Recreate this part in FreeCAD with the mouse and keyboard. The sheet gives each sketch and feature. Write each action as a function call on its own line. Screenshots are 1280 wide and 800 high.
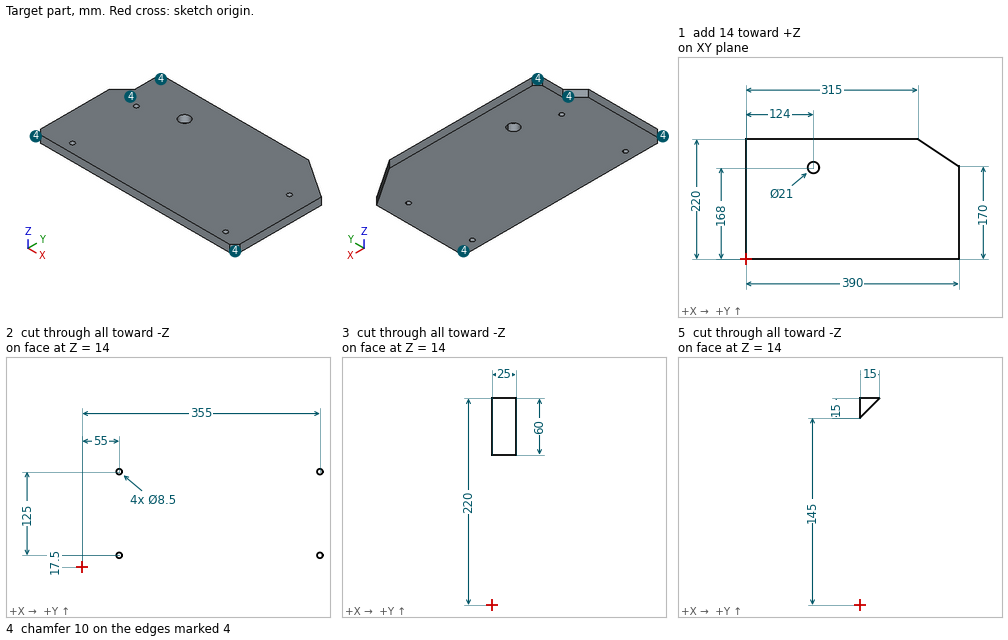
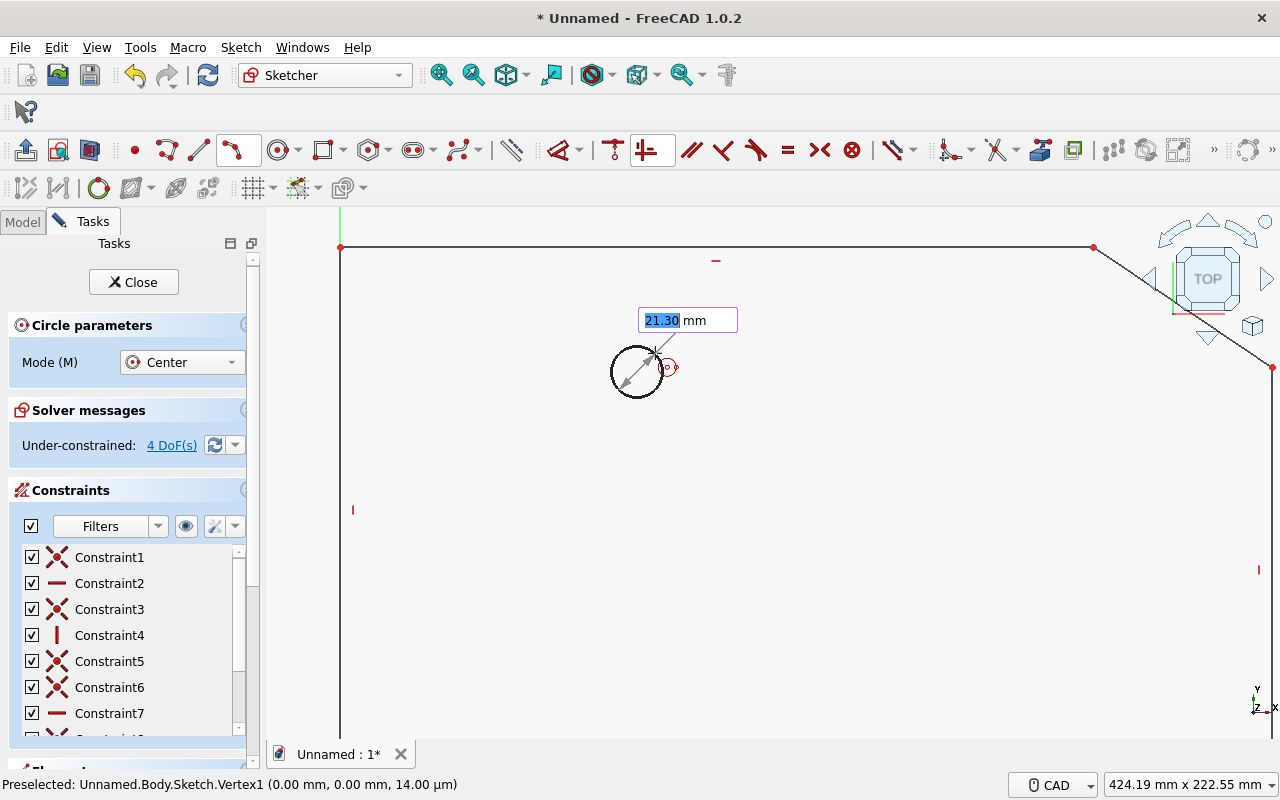
text(21)
key(Return)
key(Escape)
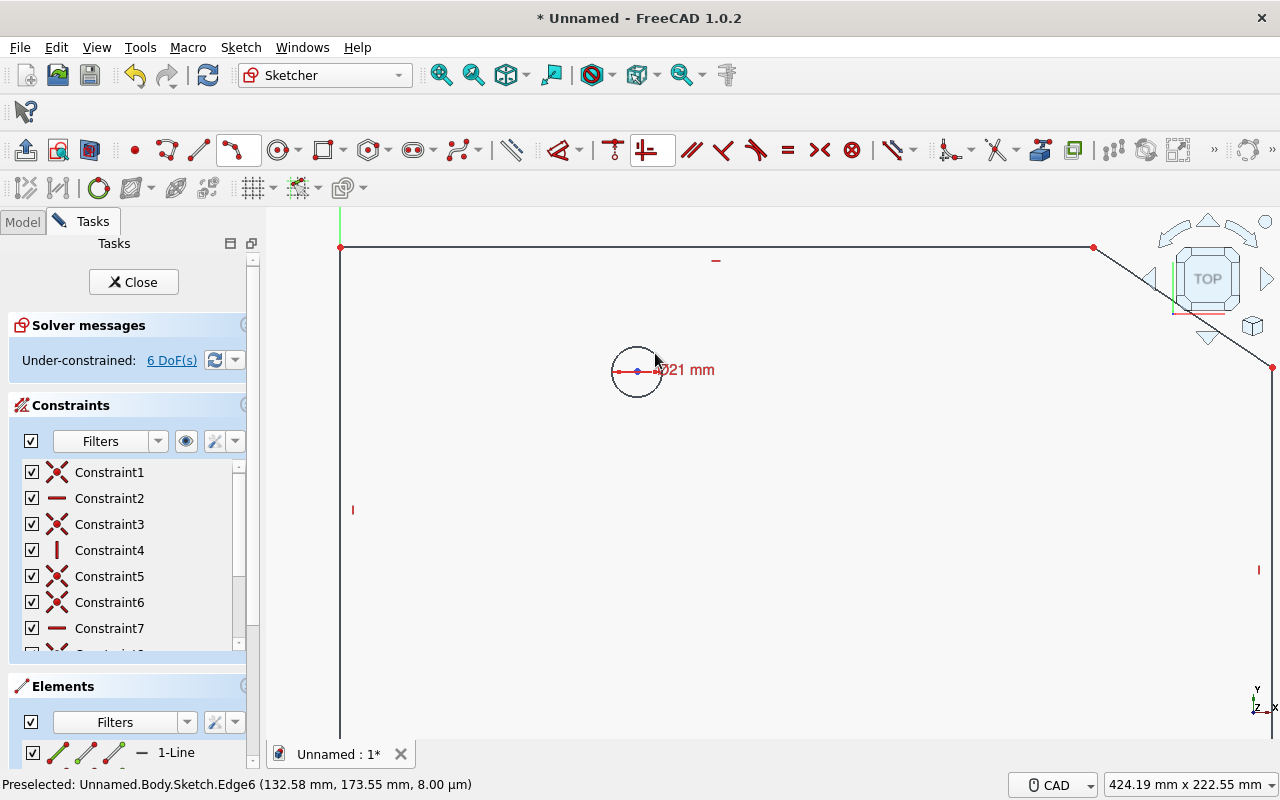
click(558, 150)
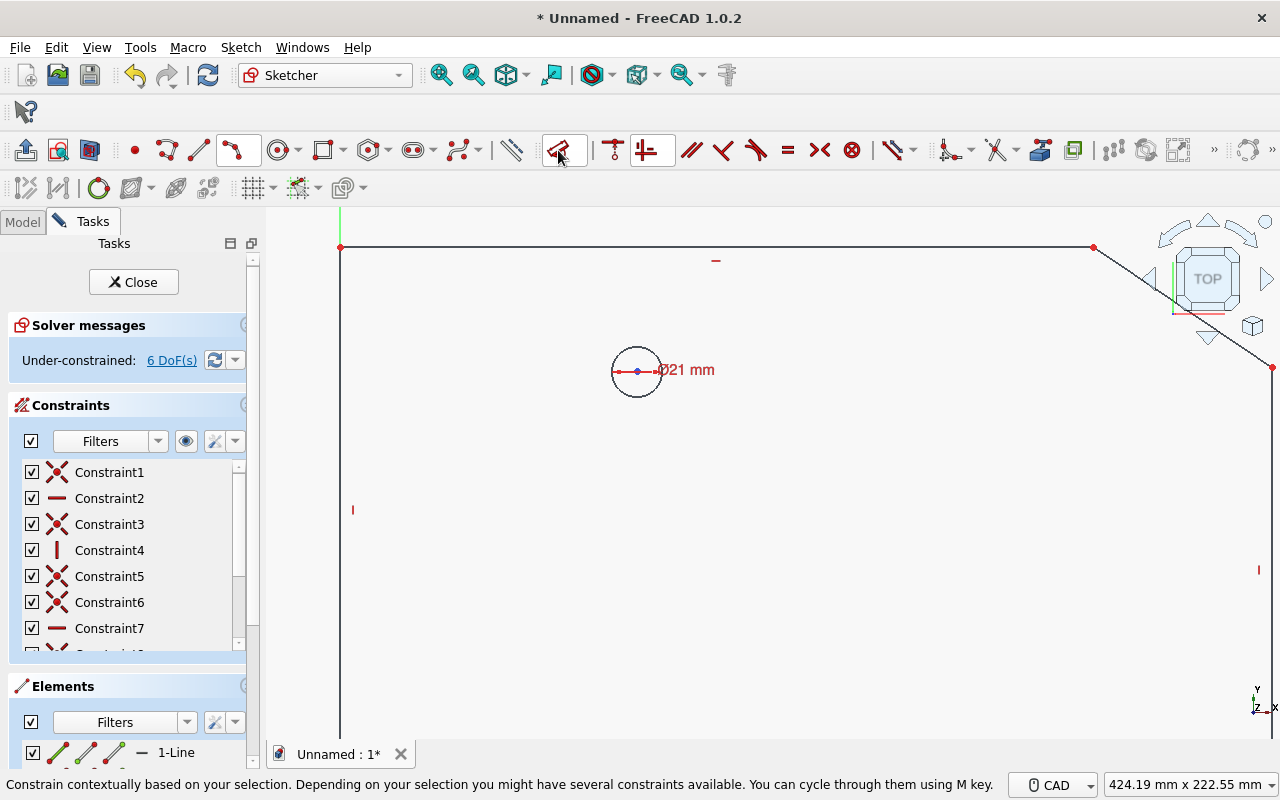
scroll(497, 399, down, 2)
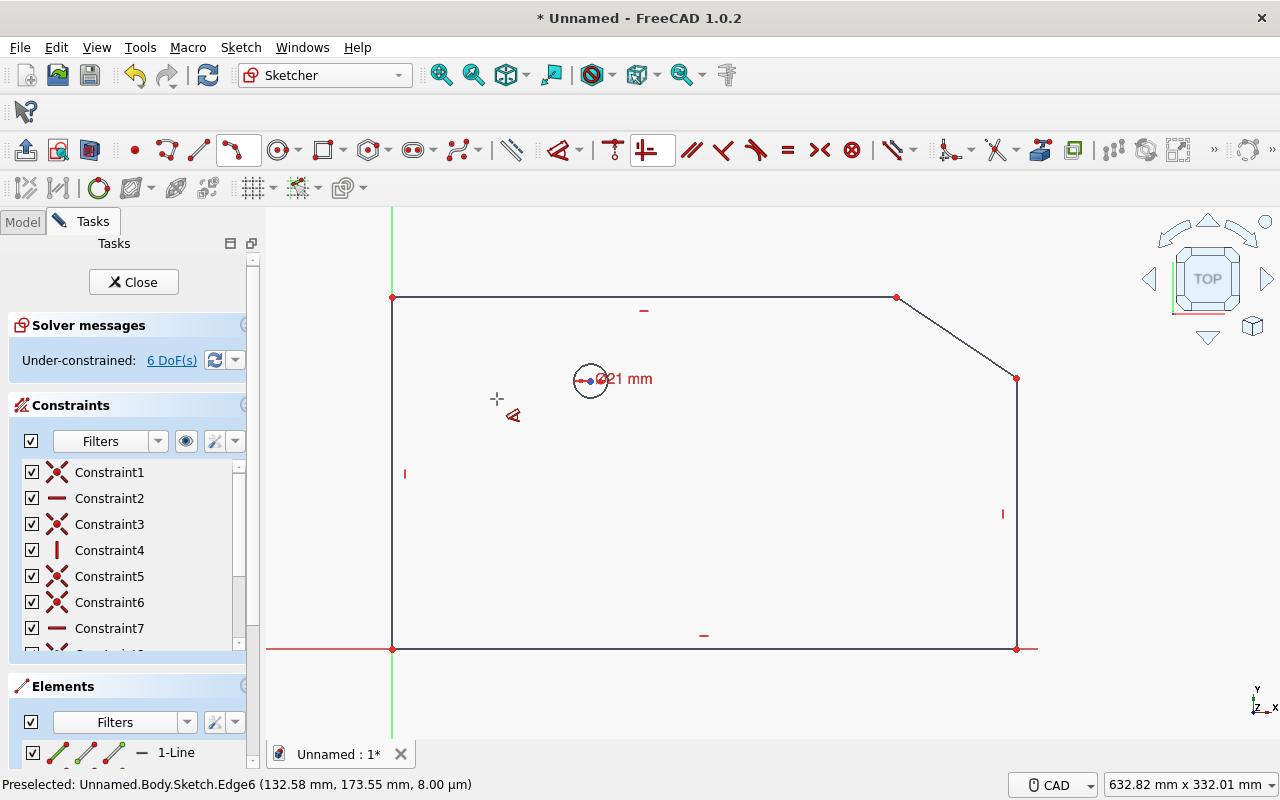
click(580, 649)
click(704, 683)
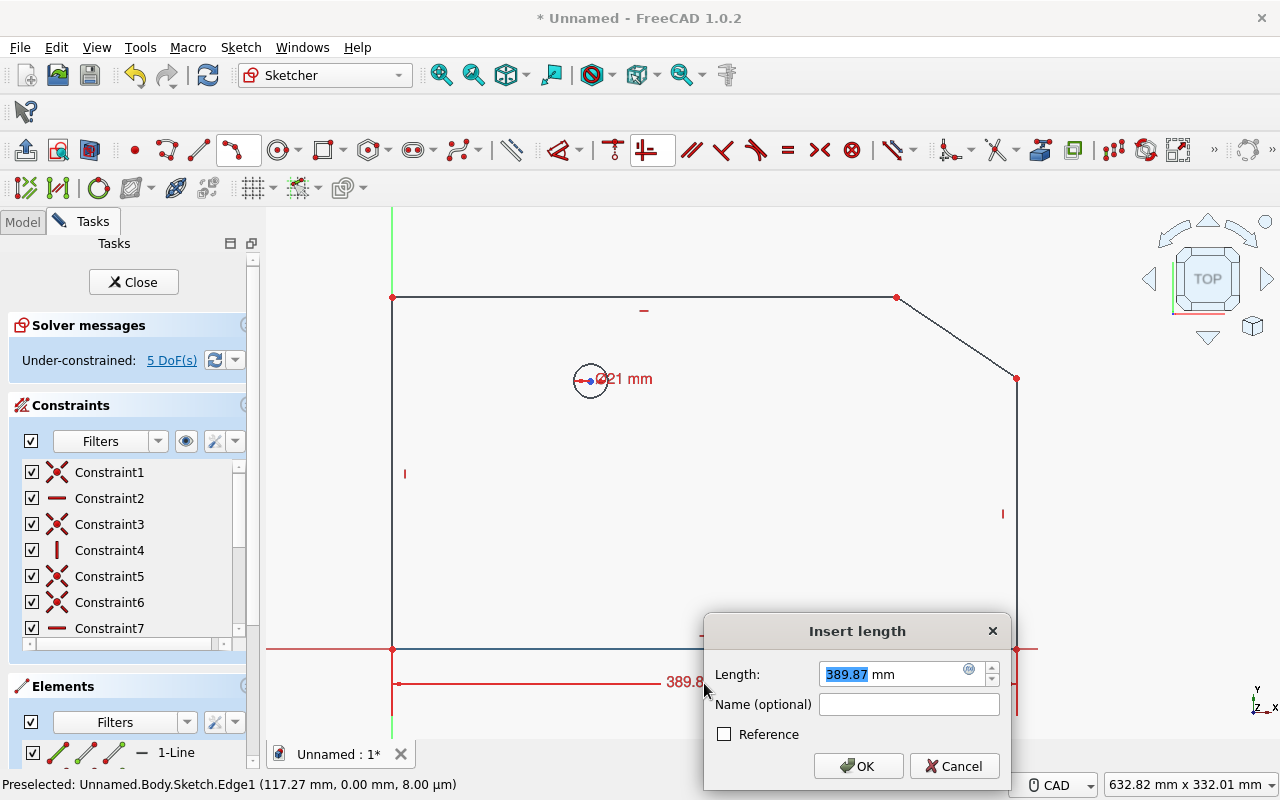
text(390)
key(Return)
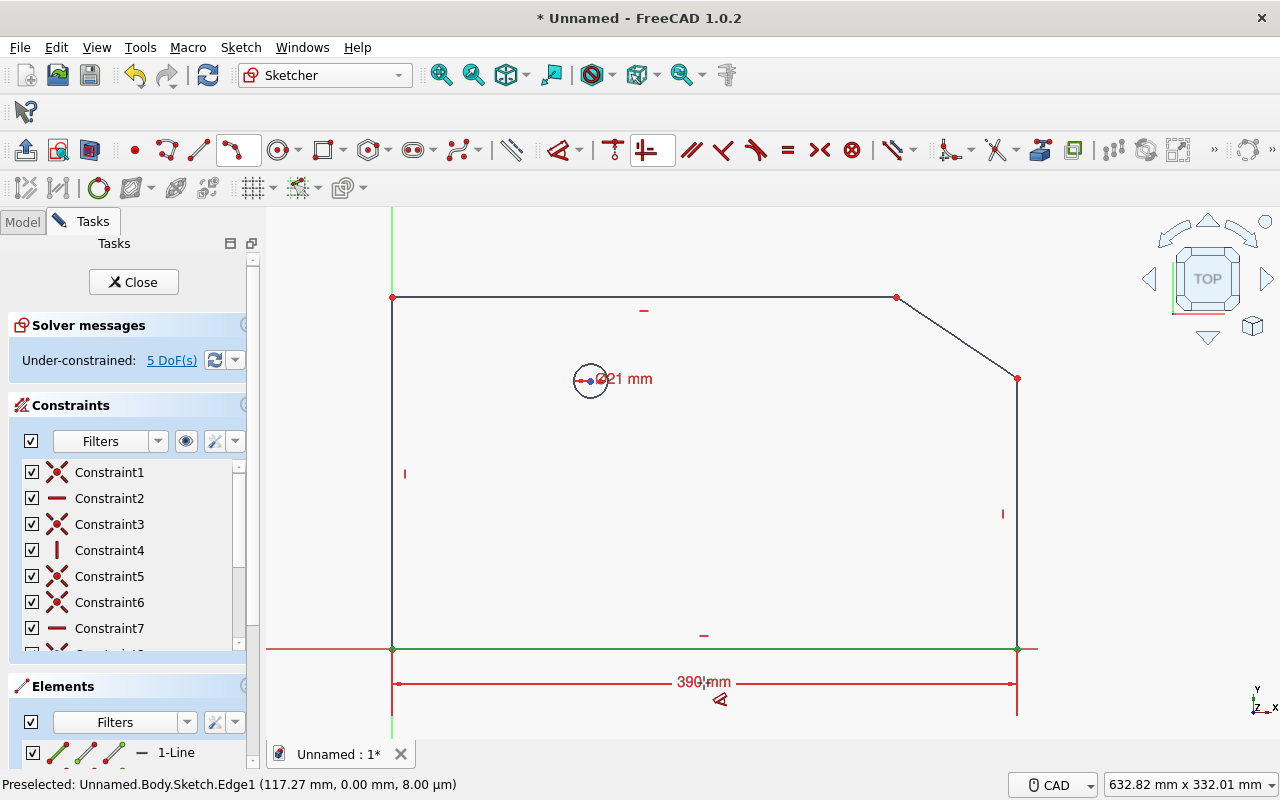
click(1017, 568)
click(1051, 514)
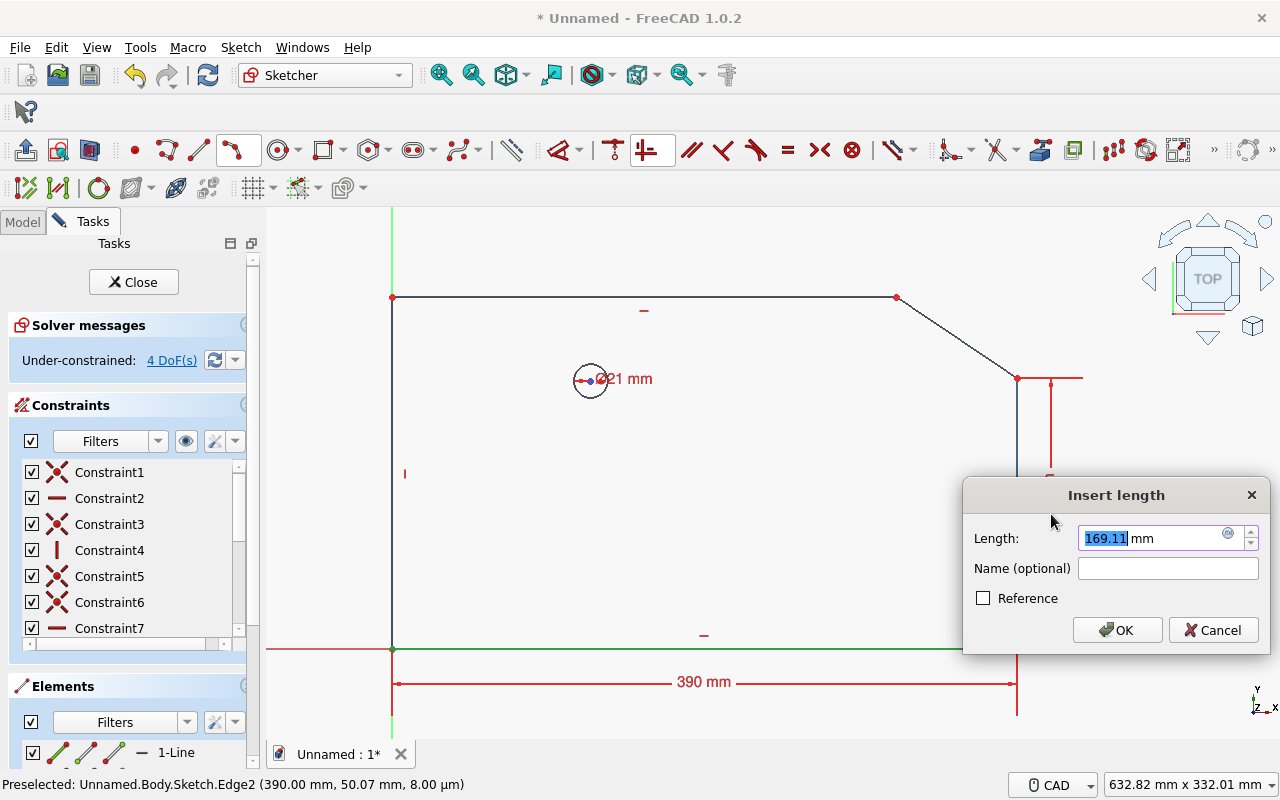
text(170)
key(Return)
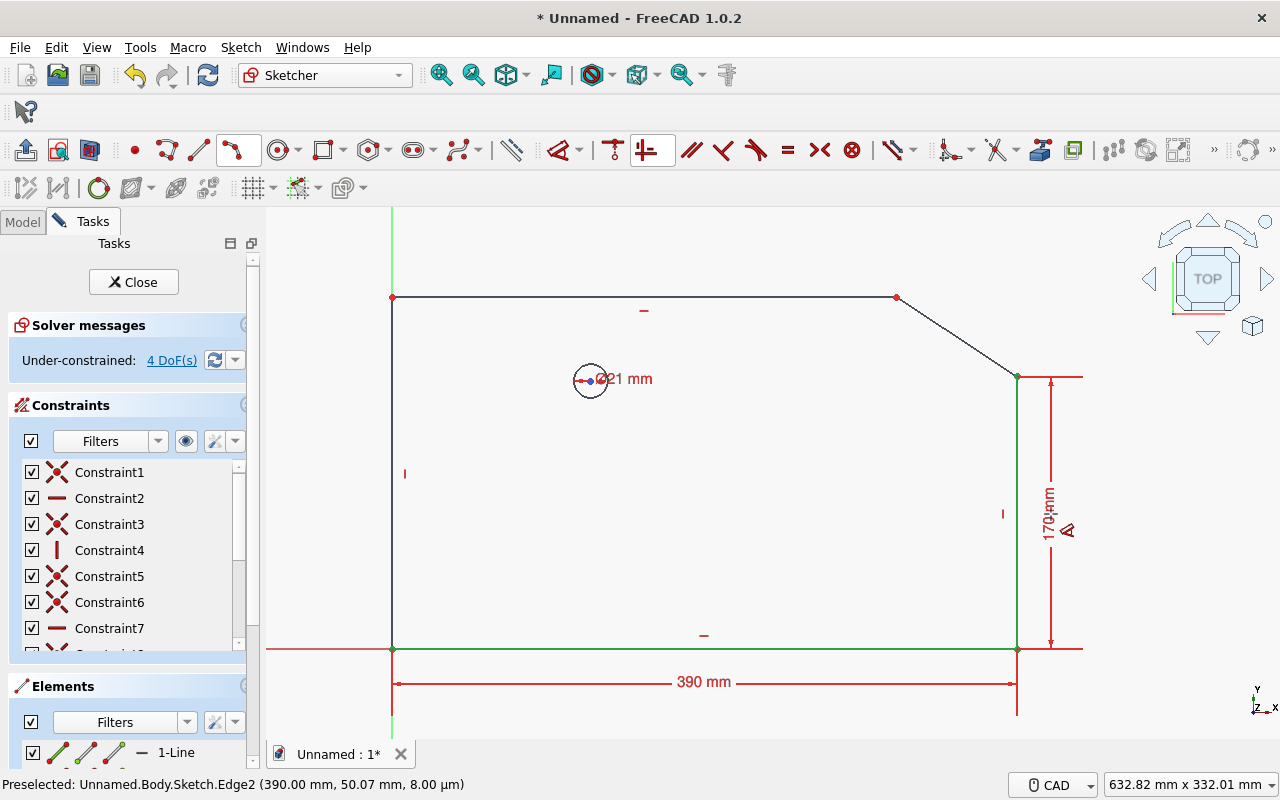
click(745, 297)
click(644, 263)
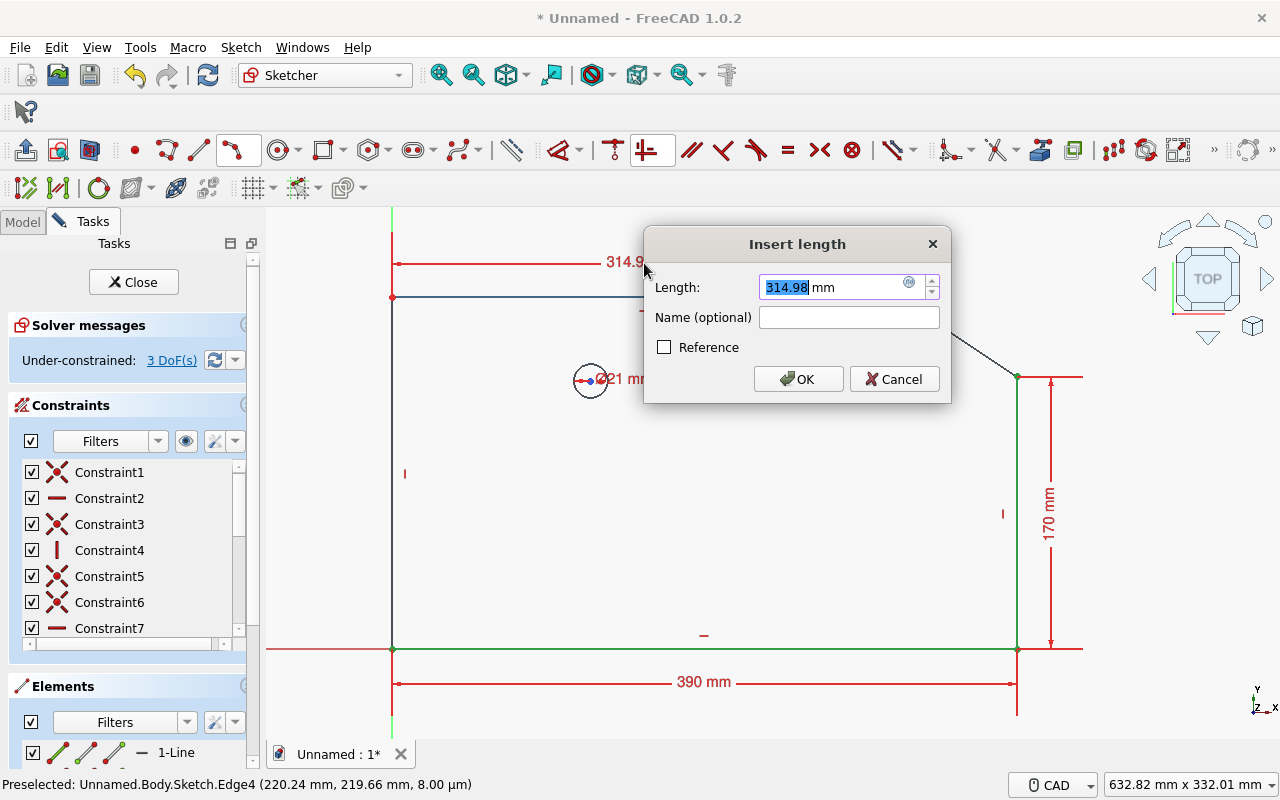
text(315)
key(Return)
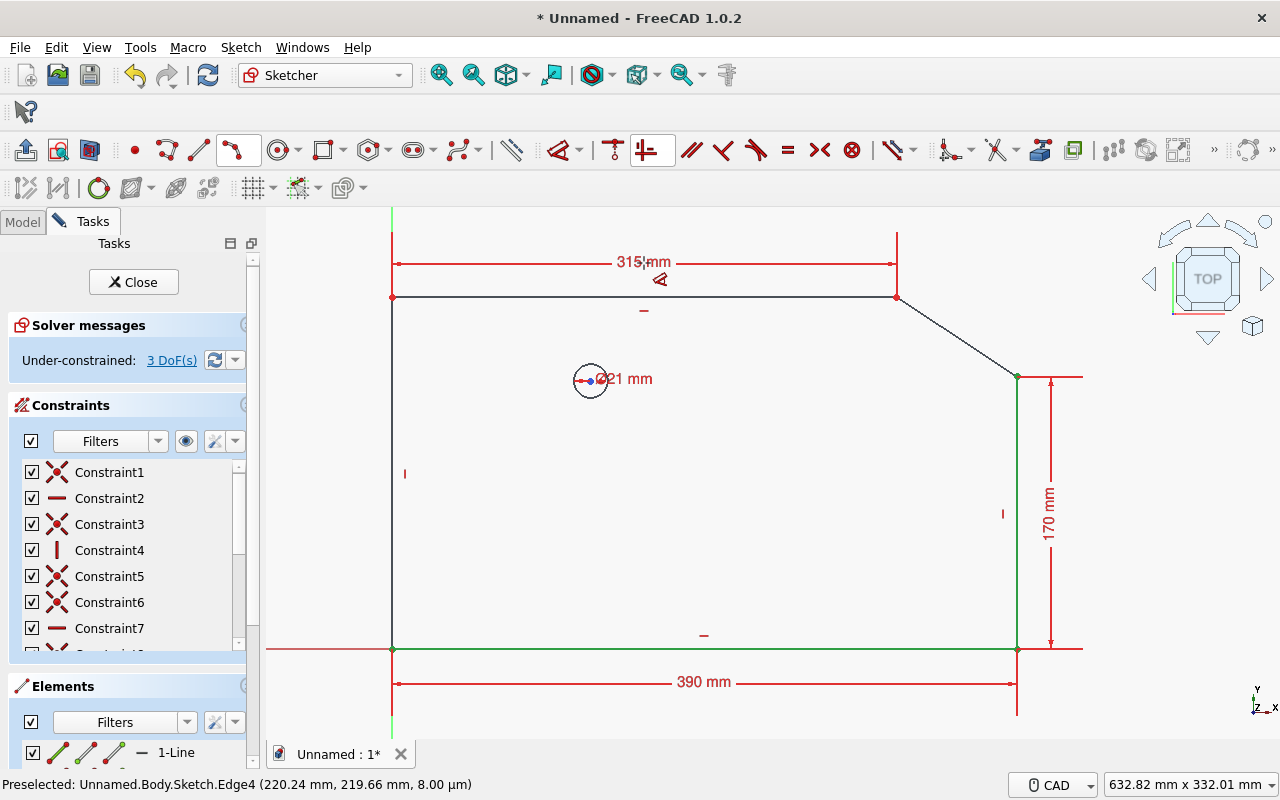
click(392, 403)
click(358, 473)